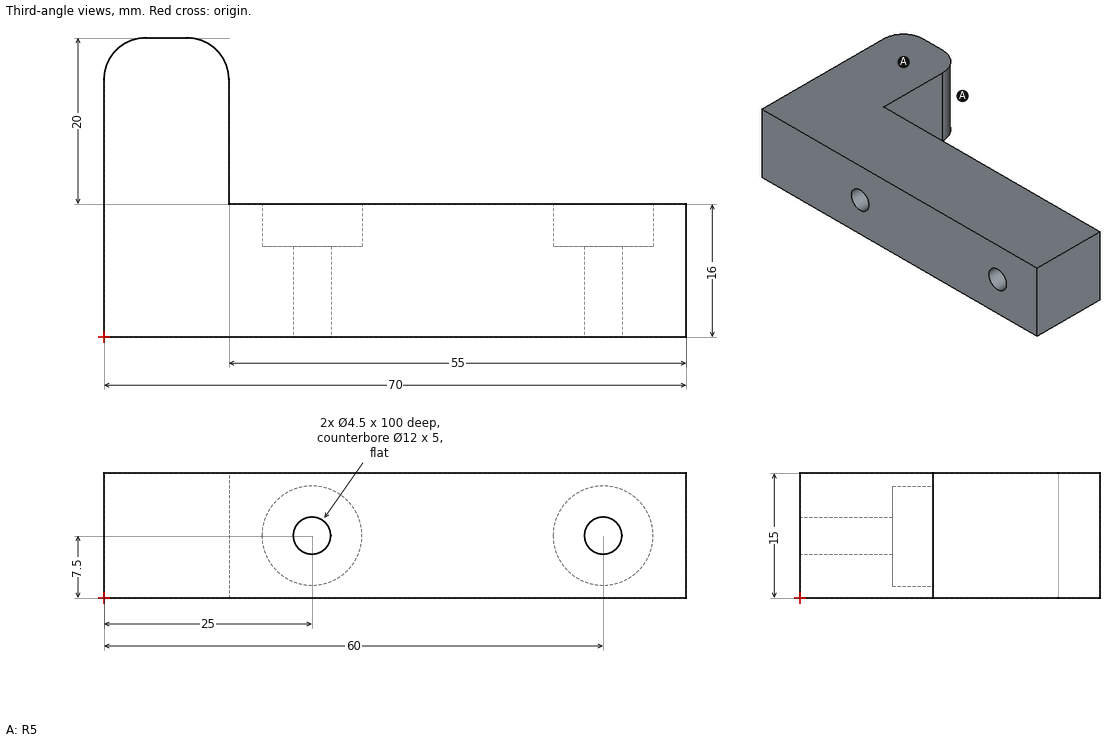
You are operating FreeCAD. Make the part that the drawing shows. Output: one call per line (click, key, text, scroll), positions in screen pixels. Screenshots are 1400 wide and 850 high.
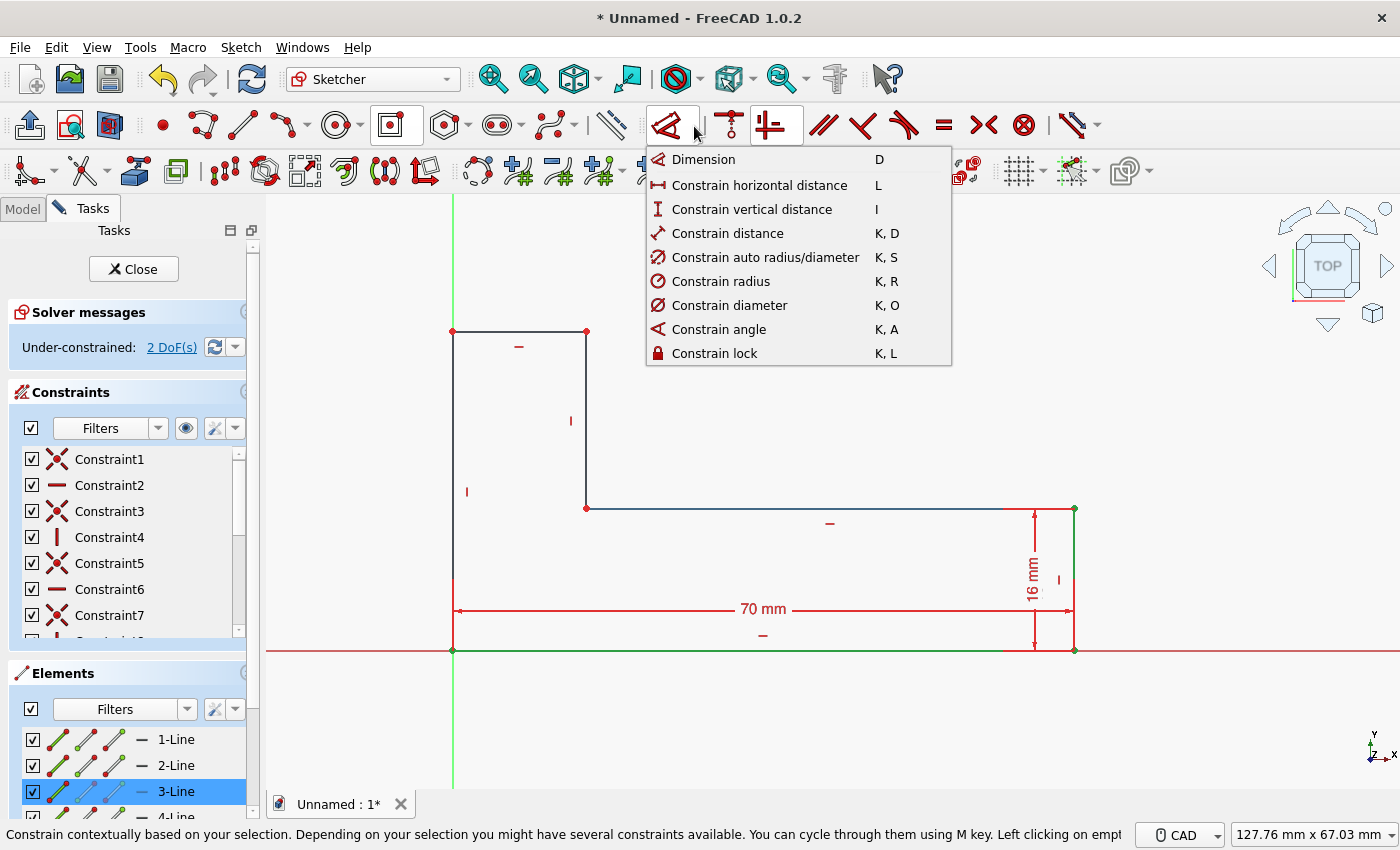
click(799, 185)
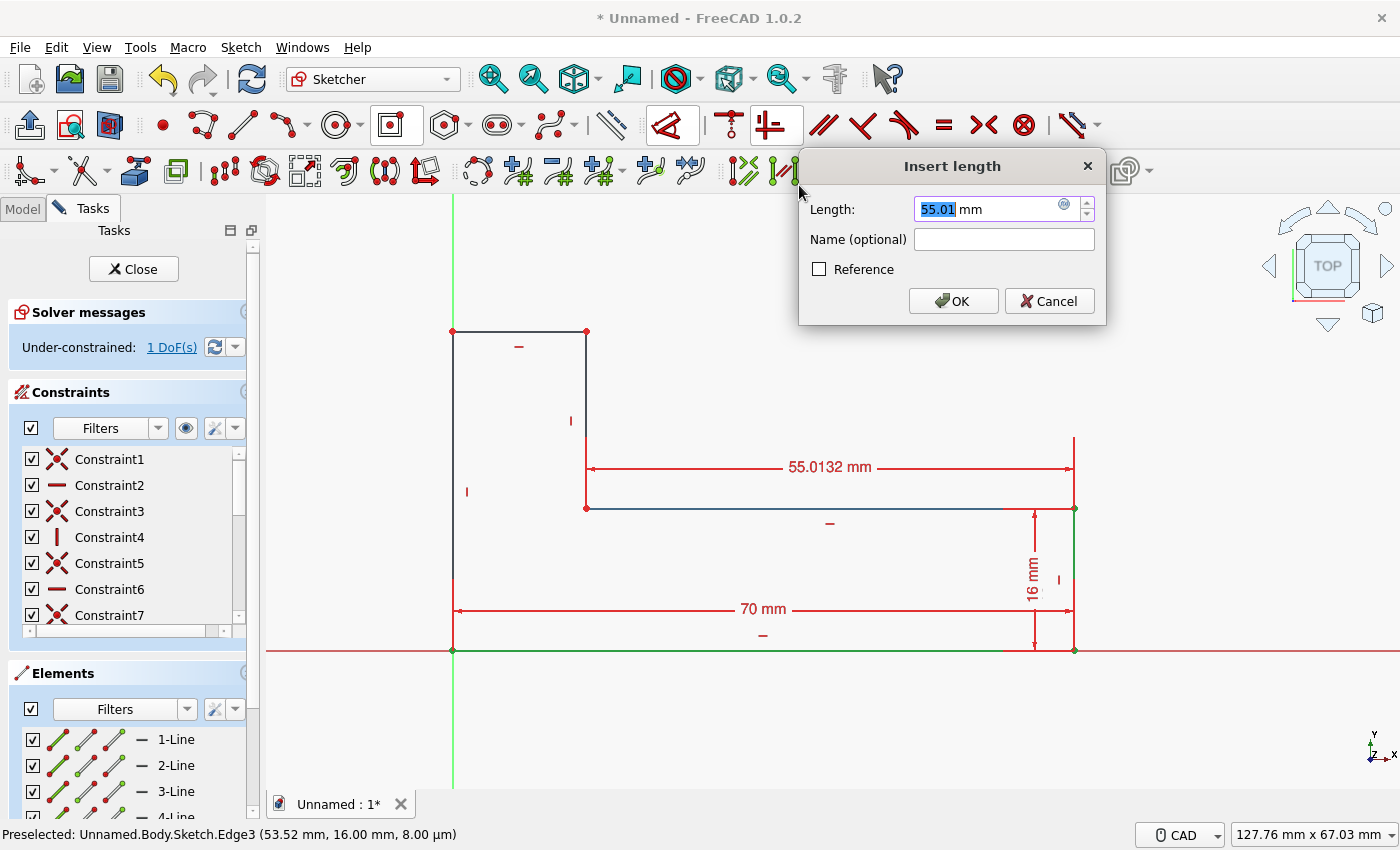
text(55)
key(Return)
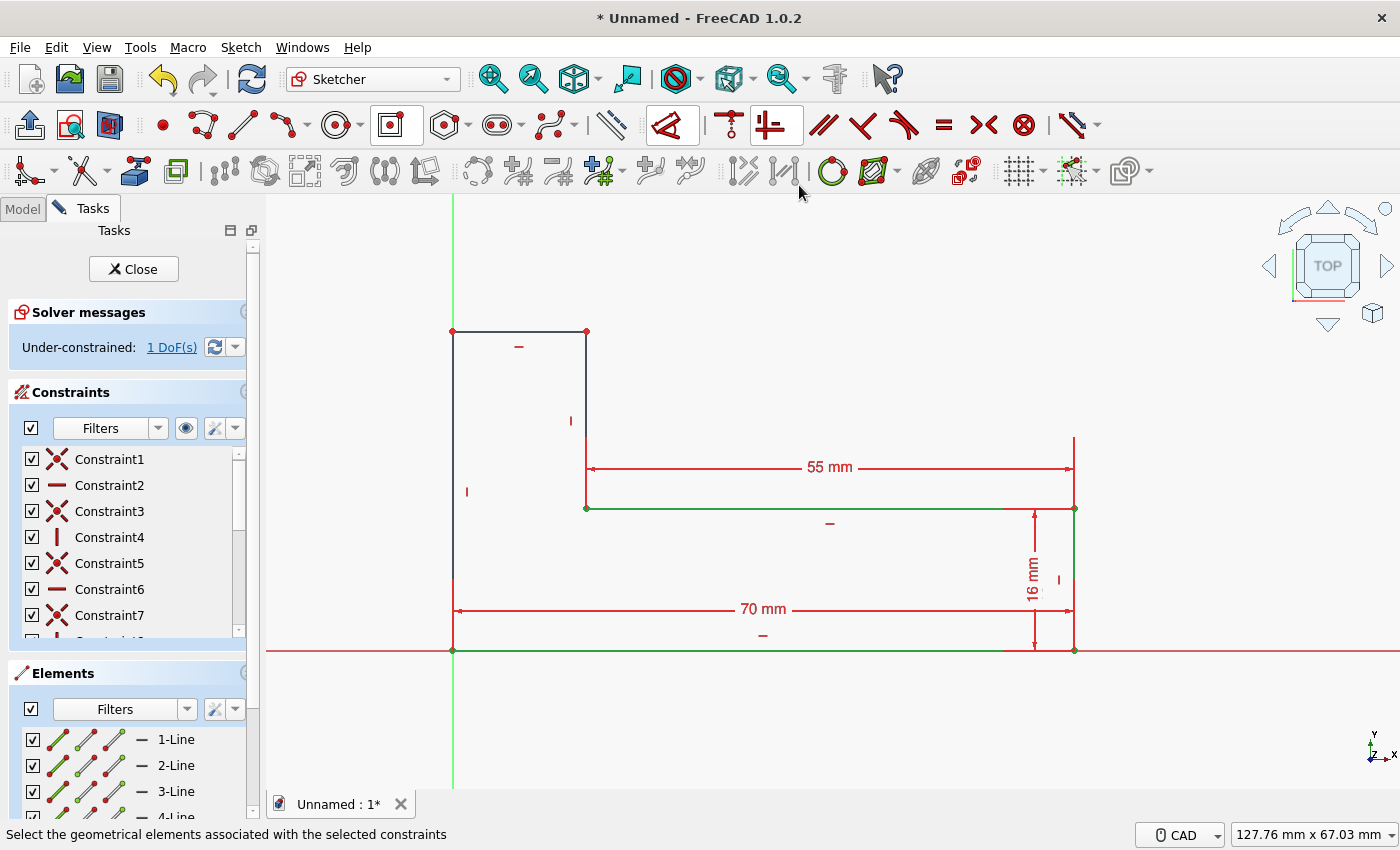
click(586, 456)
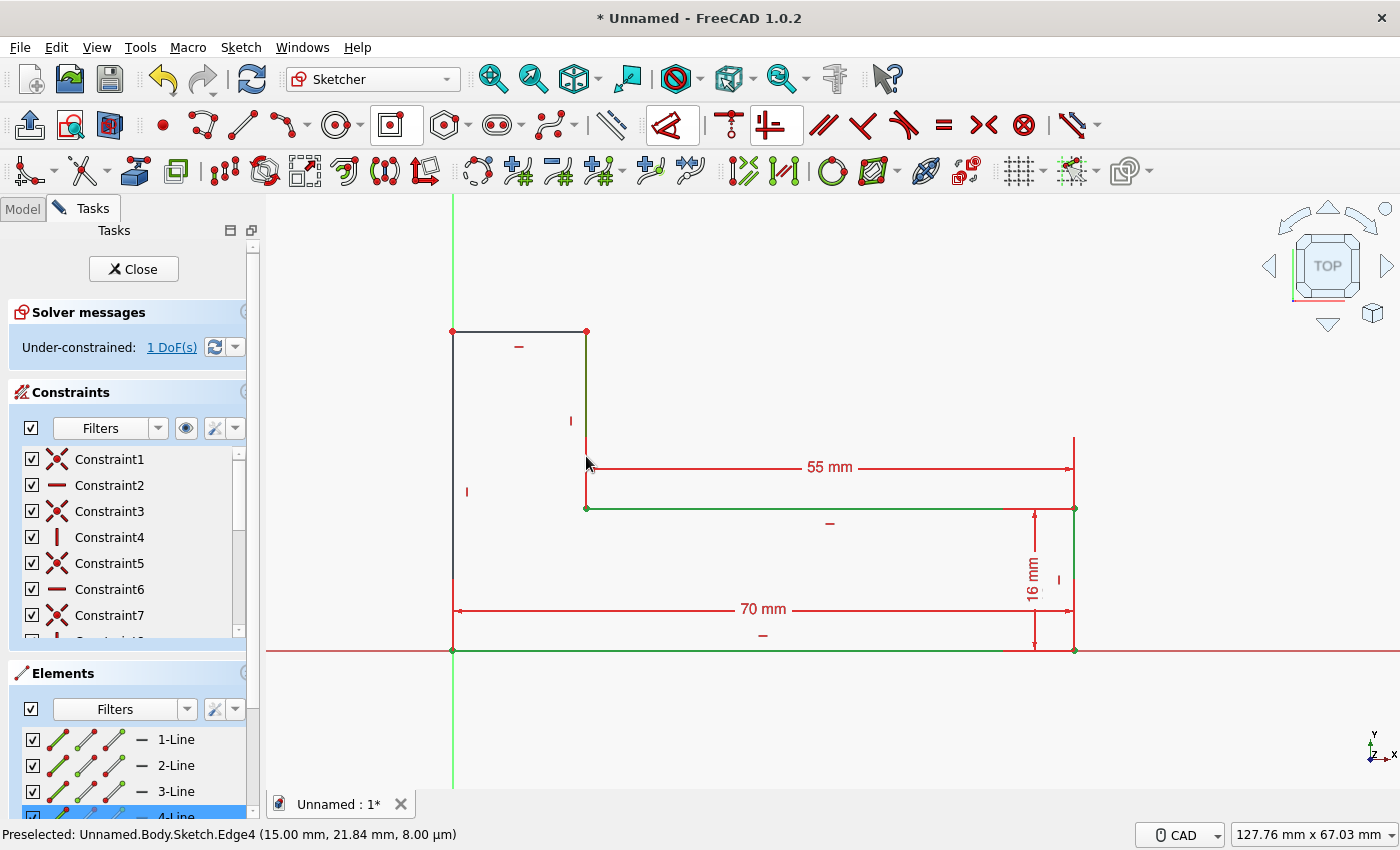
key(i)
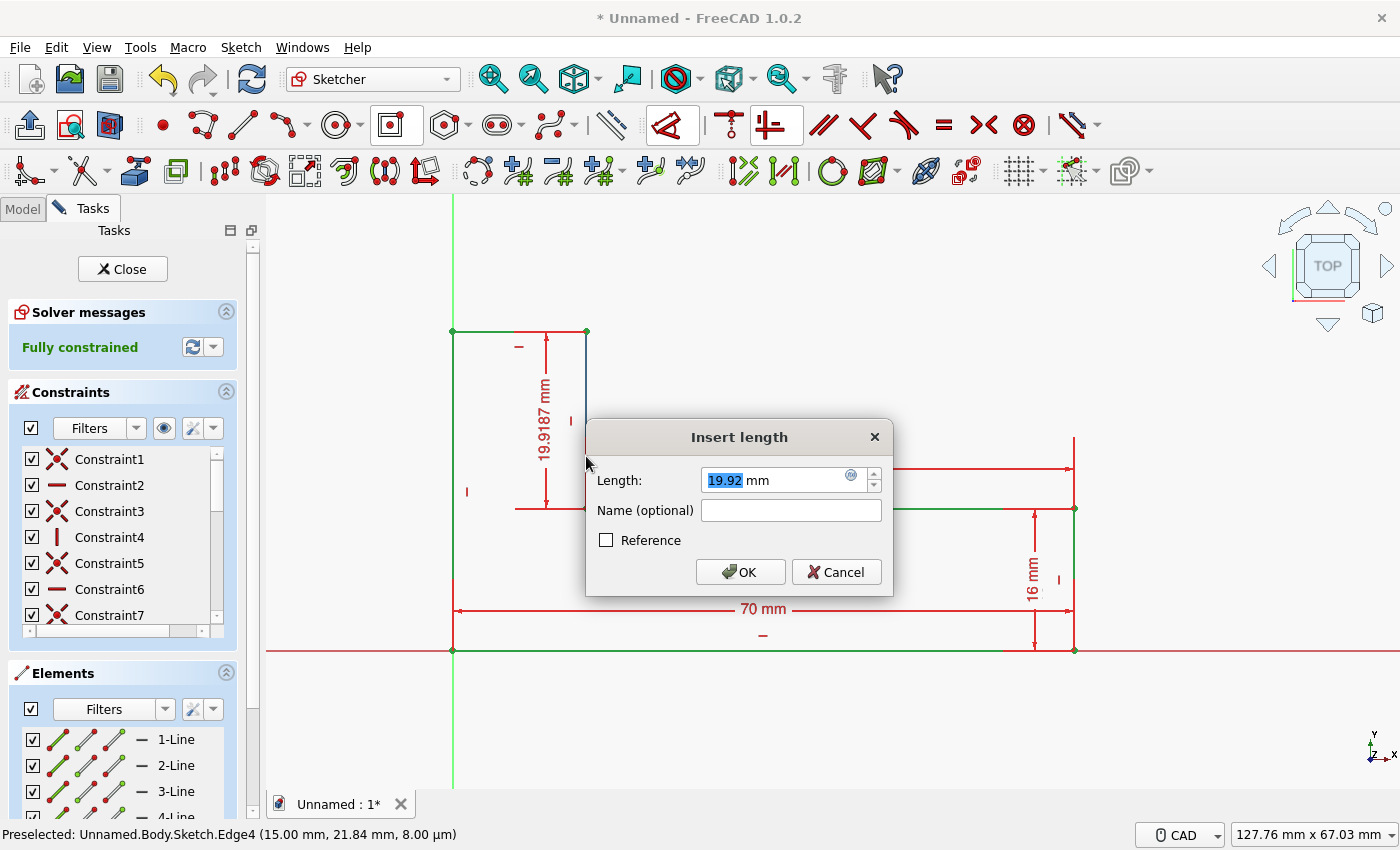
text(20)
key(Return)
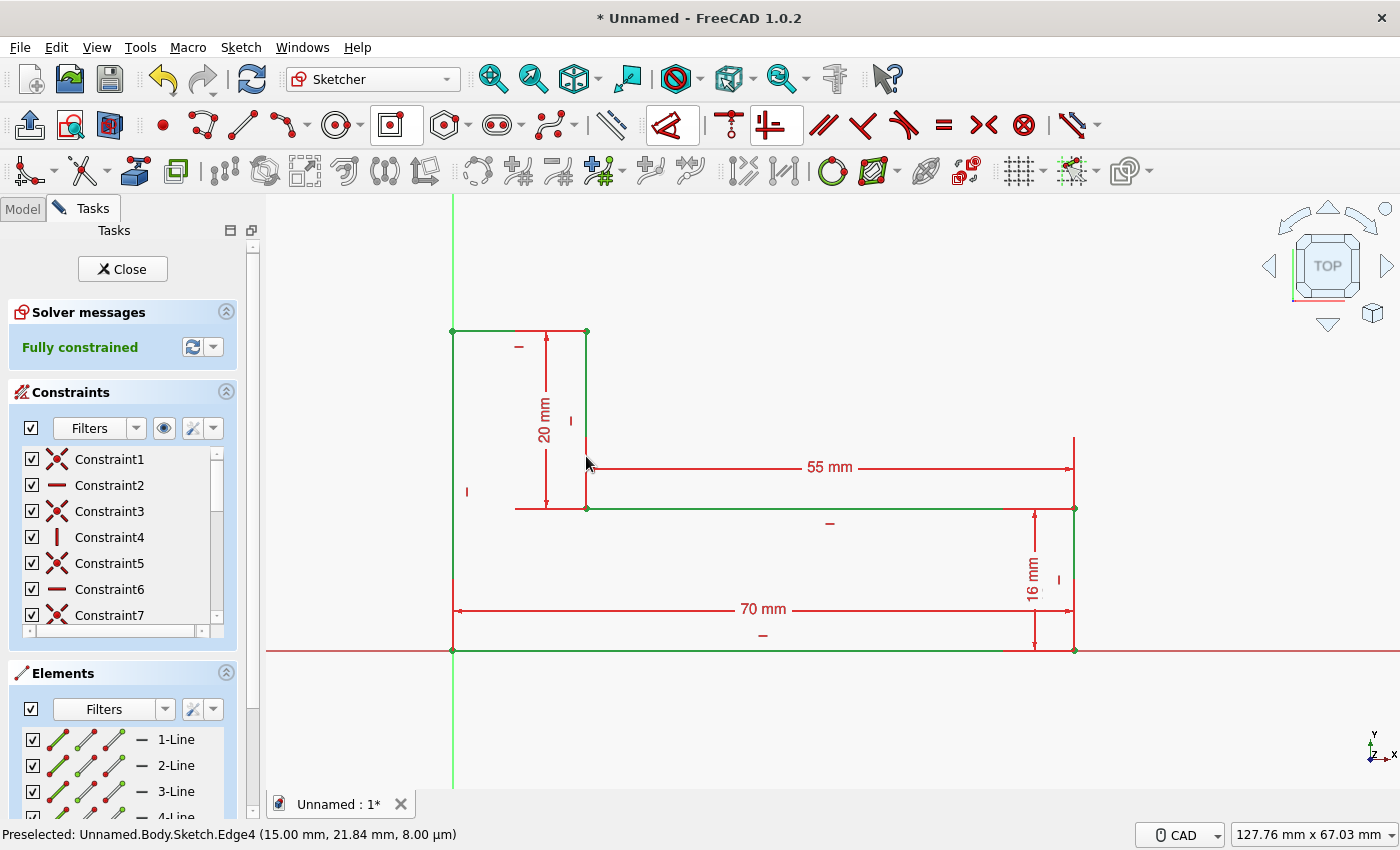
click(123, 269)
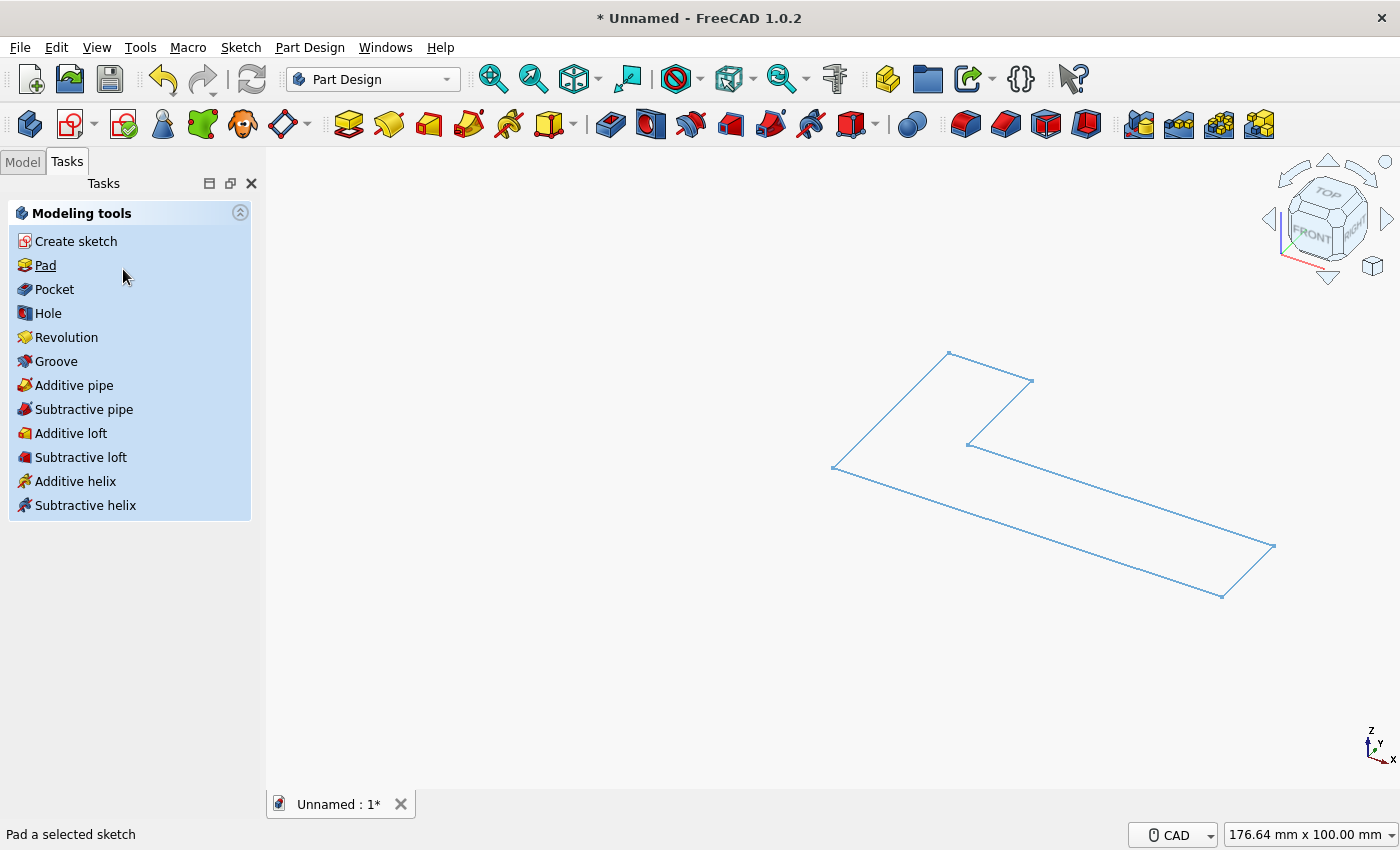
click(350, 124)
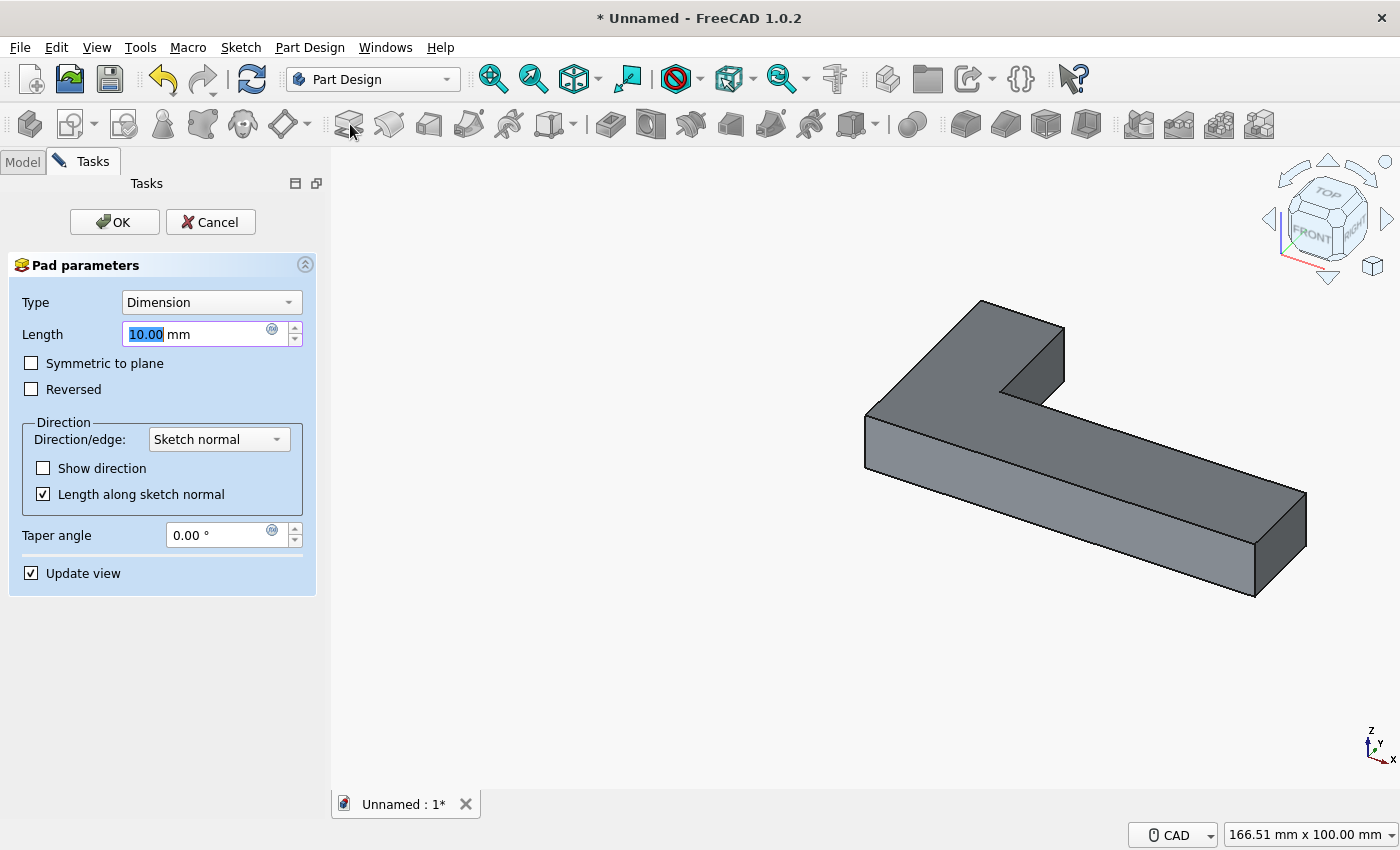
text(15)
key(Tab)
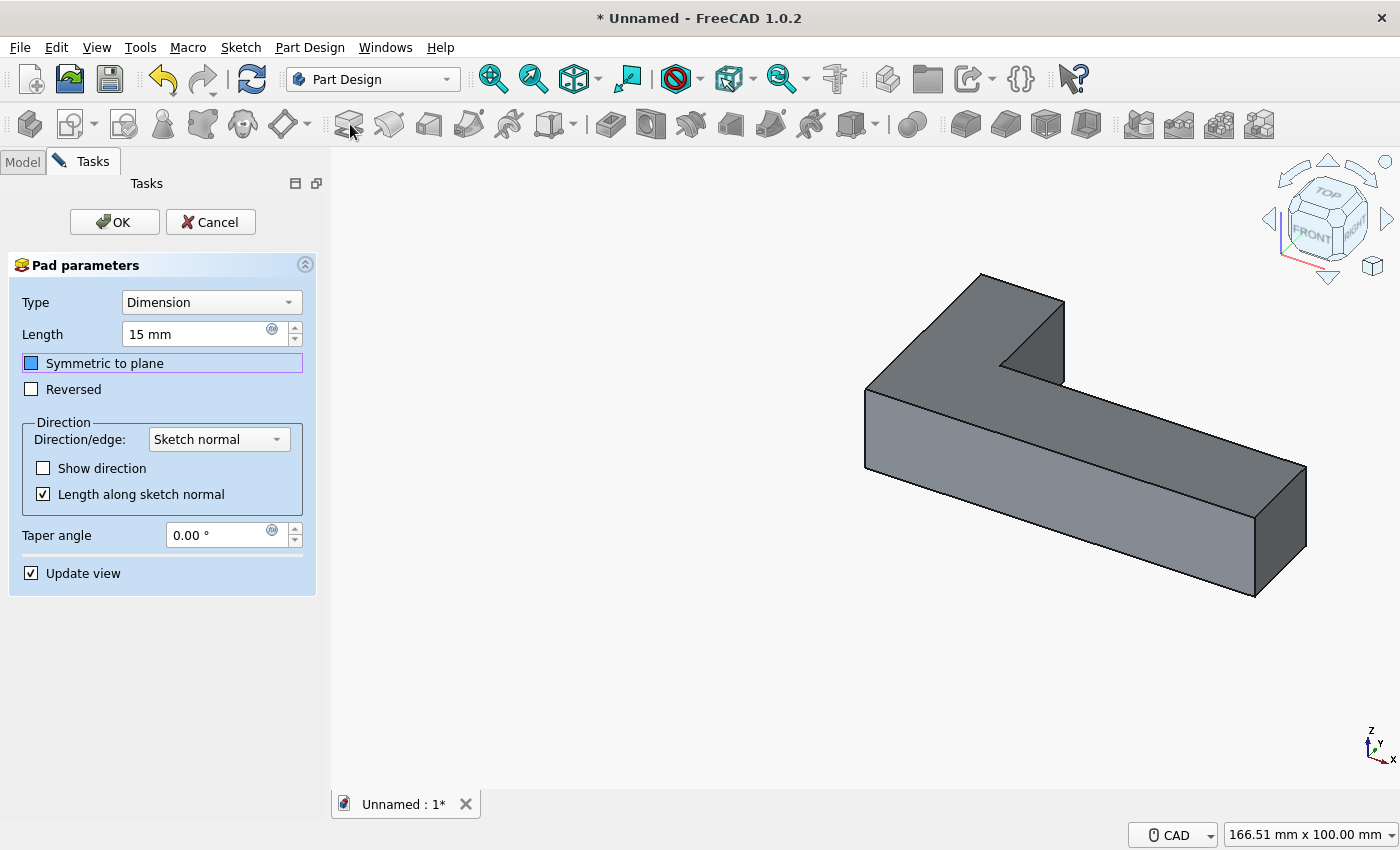
click(115, 222)